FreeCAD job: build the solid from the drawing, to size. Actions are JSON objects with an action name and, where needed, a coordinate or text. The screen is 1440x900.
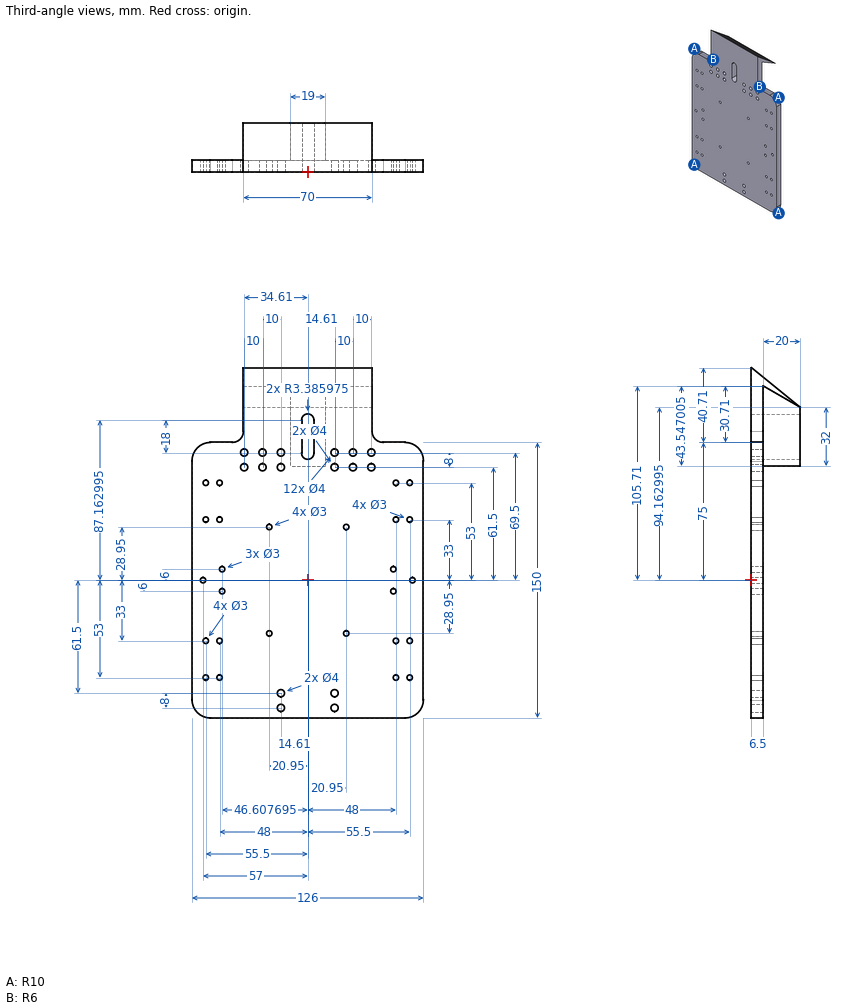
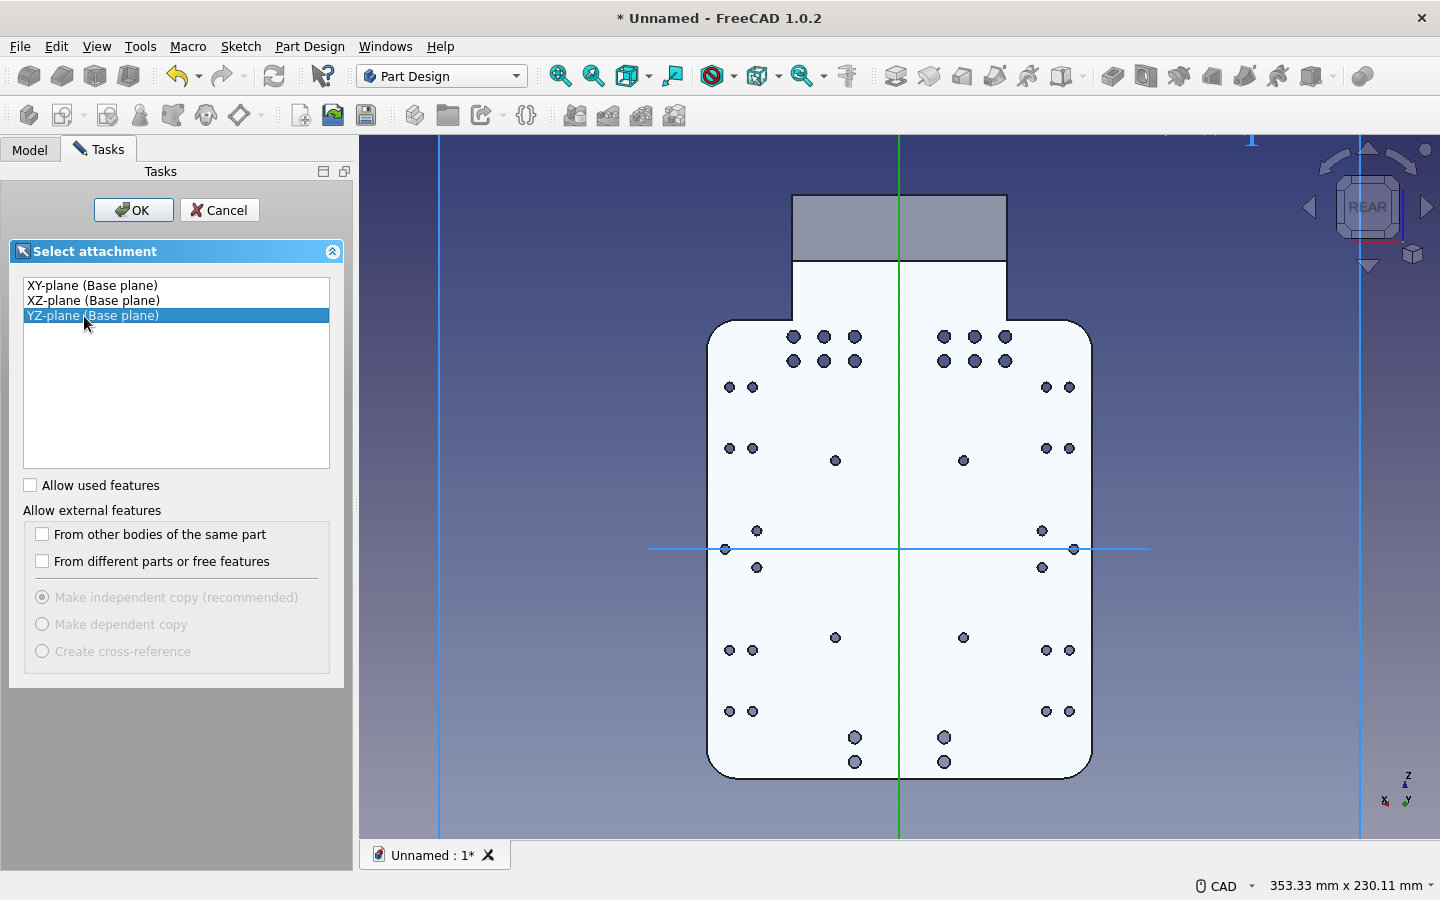
{"action": "left_click", "coordinate": [134, 210]}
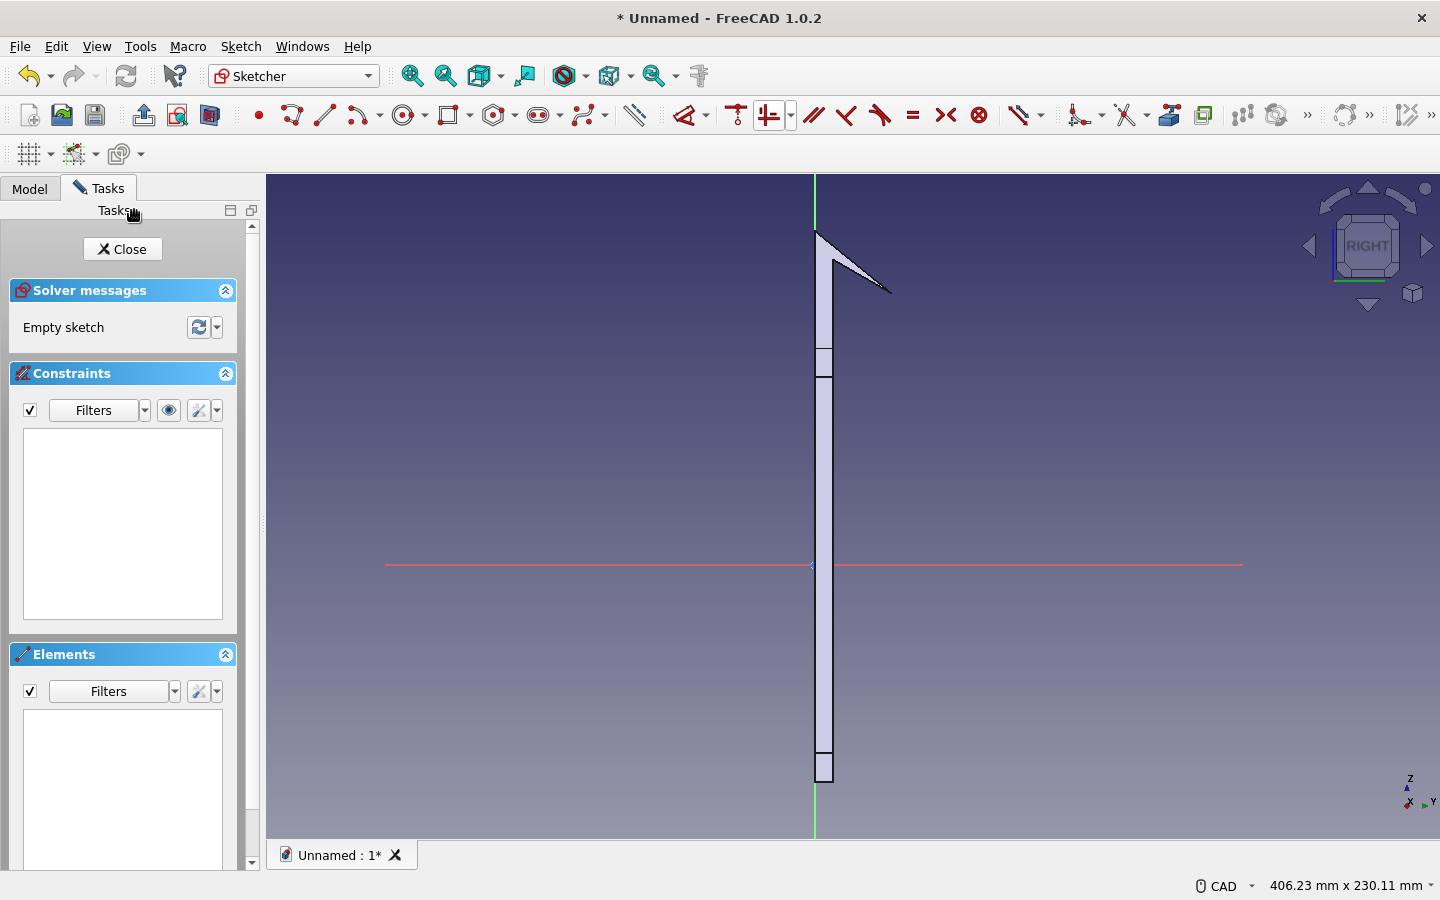
{"action": "left_click", "coordinate": [210, 116]}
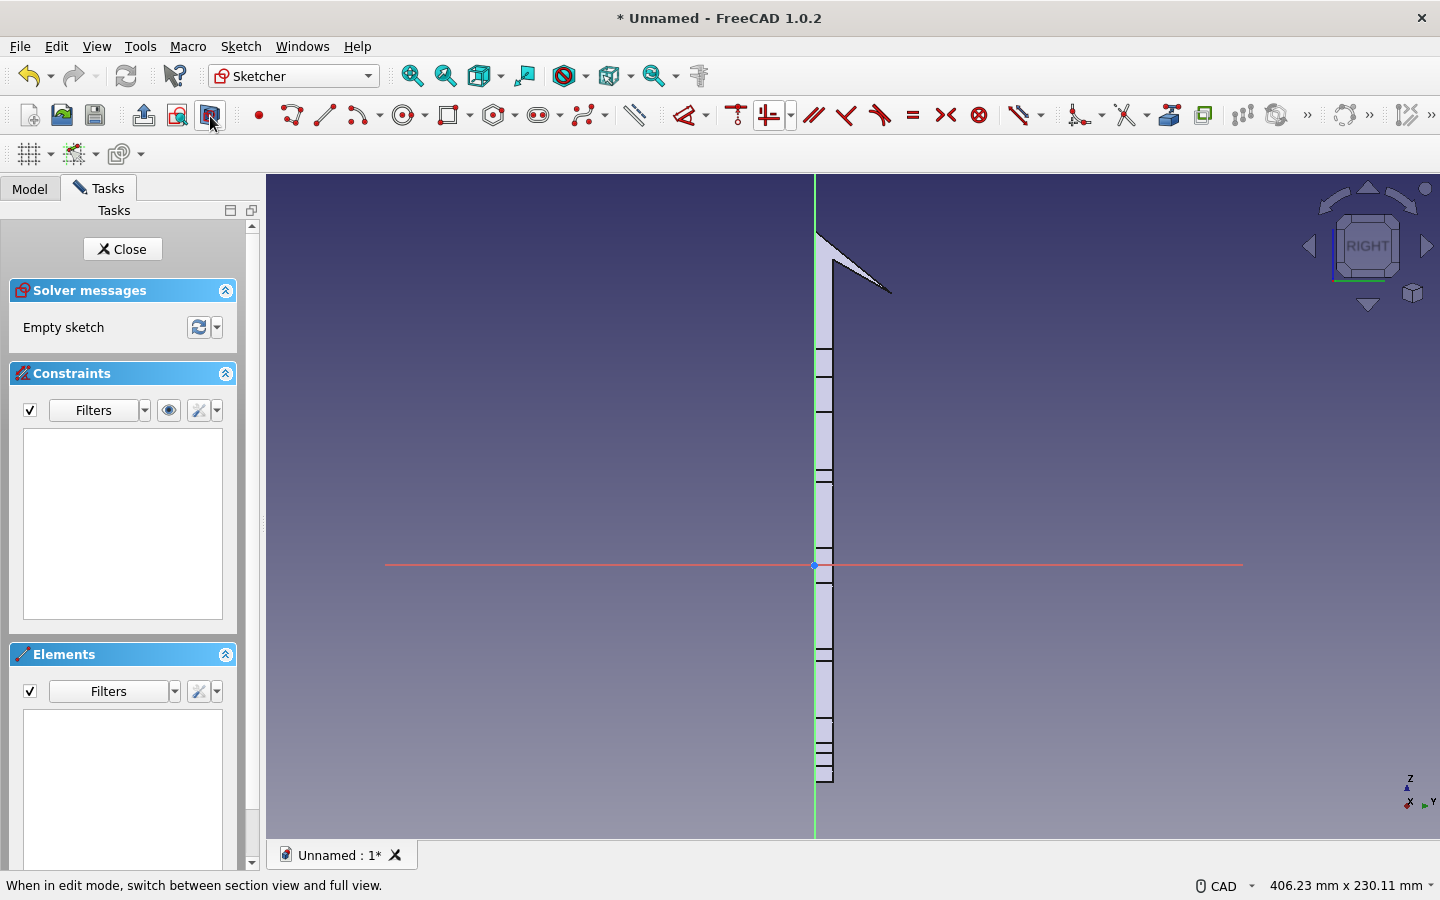
{"action": "scroll", "coordinate": [992, 222], "scroll_direction": "up", "scroll_amount": 2}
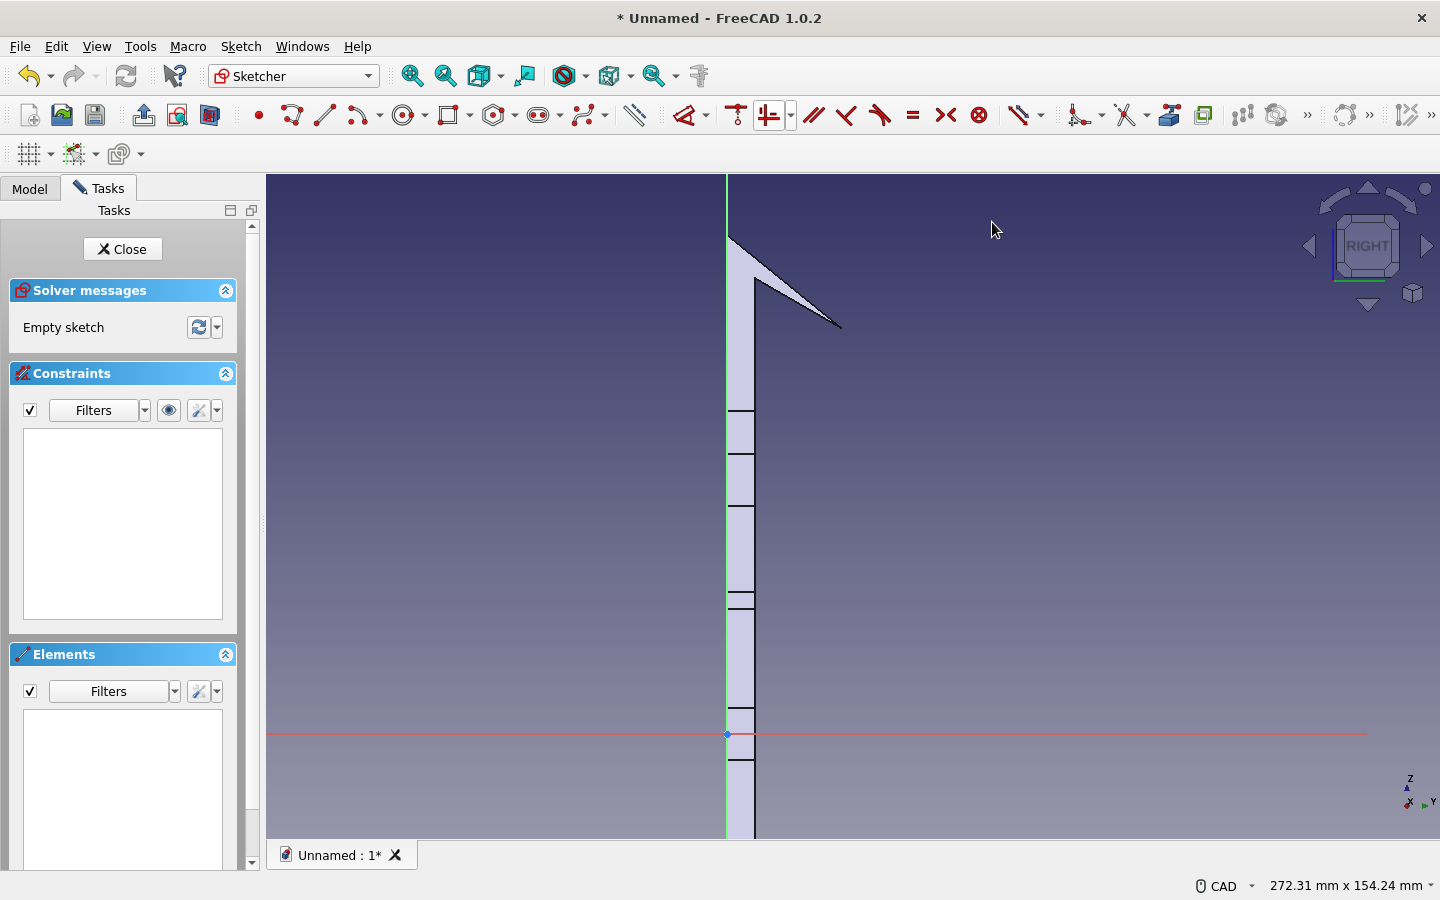
{"action": "left_click", "coordinate": [292, 116]}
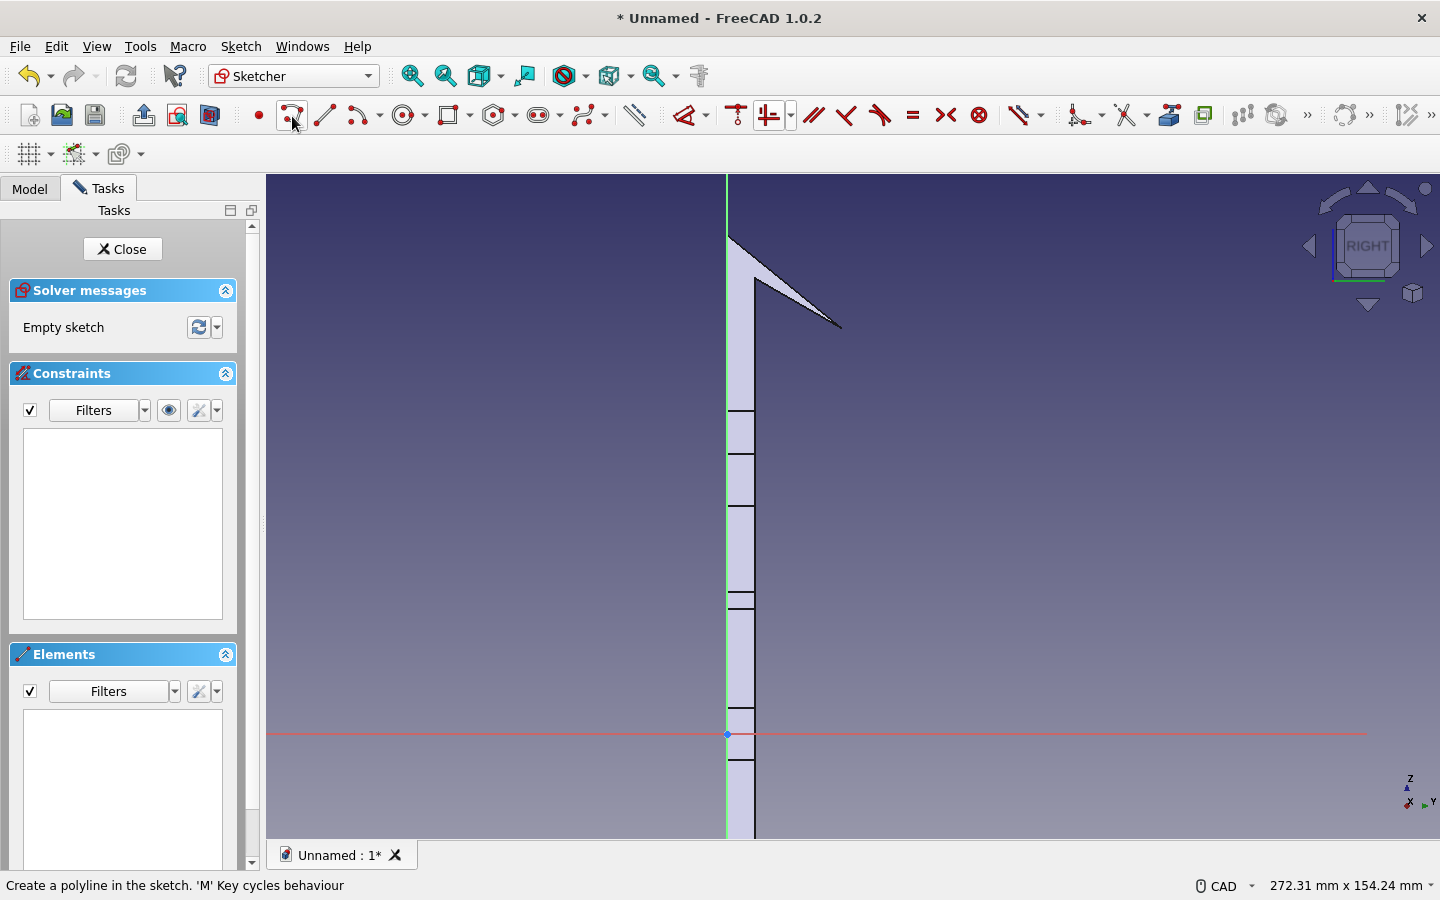
{"action": "left_click", "coordinate": [755, 466]}
{"action": "left_click", "coordinate": [841, 466]}
{"action": "left_click", "coordinate": [841, 328]}
{"action": "left_click", "coordinate": [755, 278]}
{"action": "left_click", "coordinate": [755, 467]}
{"action": "key", "text": "Escape"}
{"action": "key", "text": "Escape"}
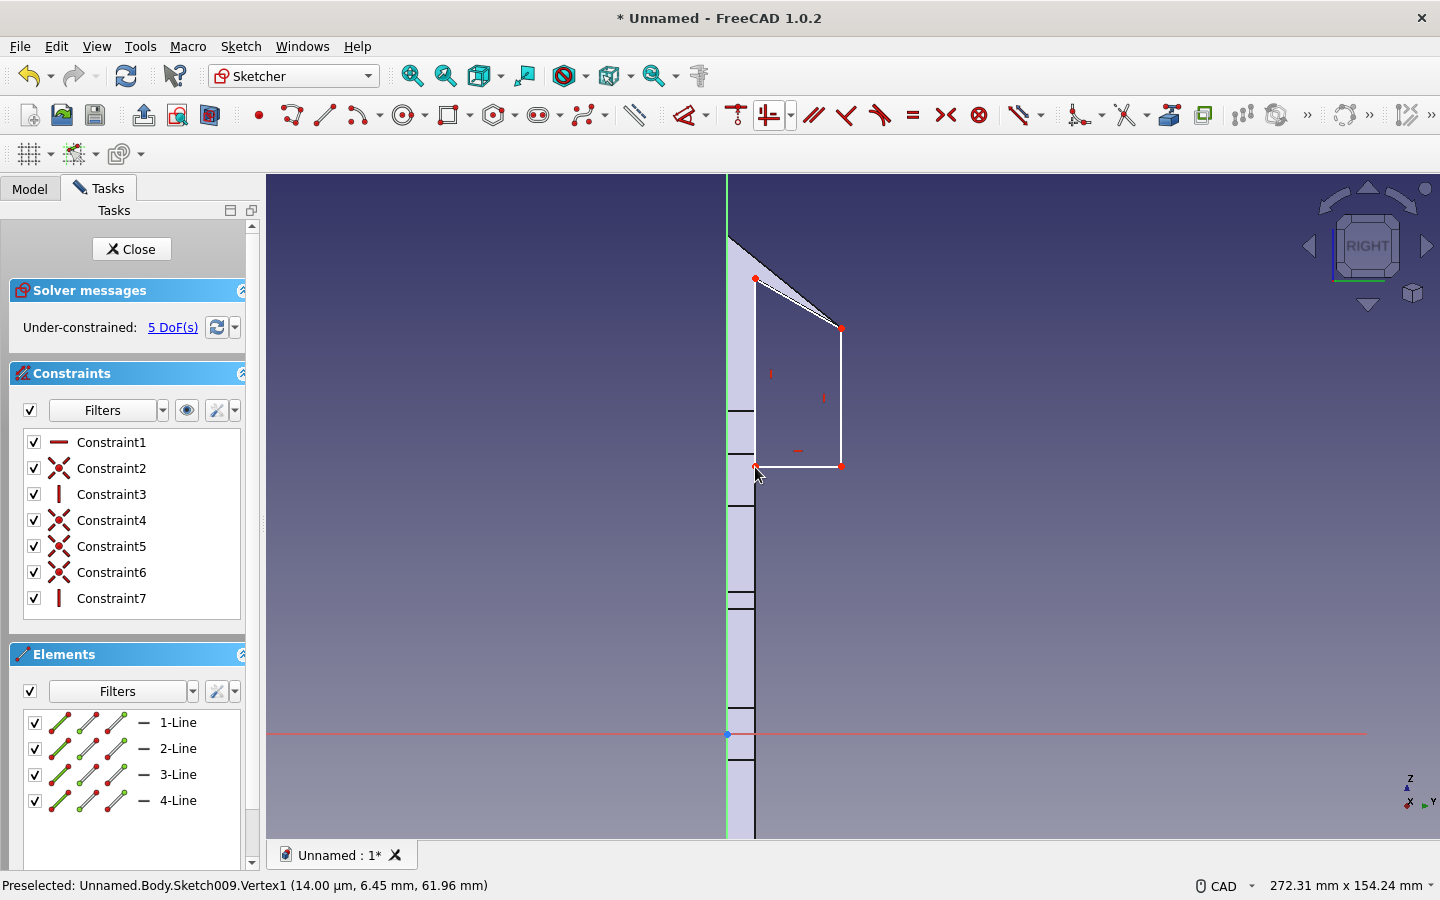
{"action": "key", "text": "d"}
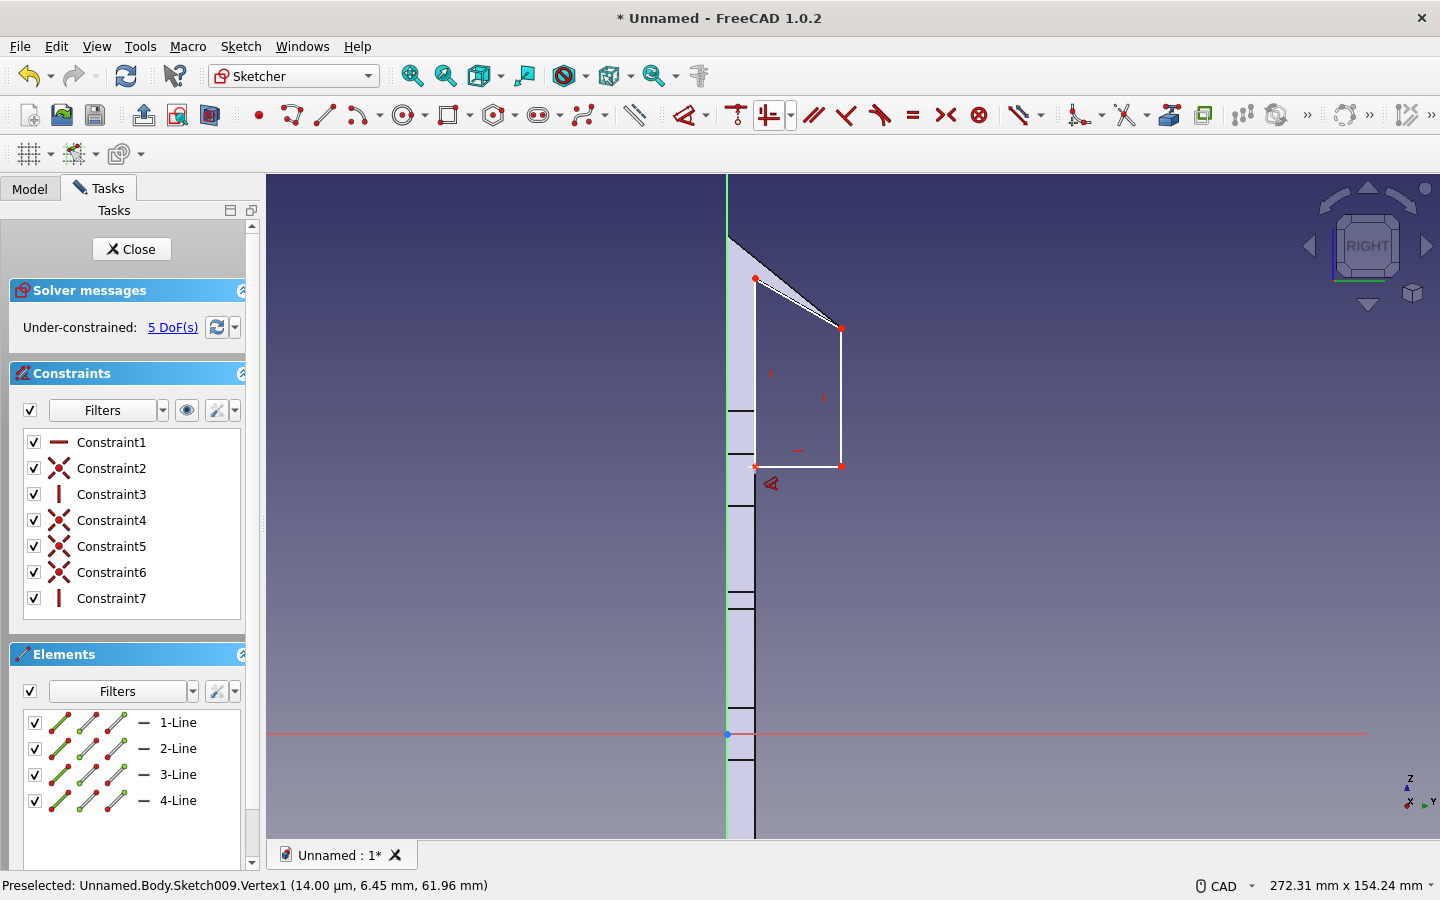
{"action": "left_click", "coordinate": [781, 467]}
{"action": "left_click", "coordinate": [798, 433]}